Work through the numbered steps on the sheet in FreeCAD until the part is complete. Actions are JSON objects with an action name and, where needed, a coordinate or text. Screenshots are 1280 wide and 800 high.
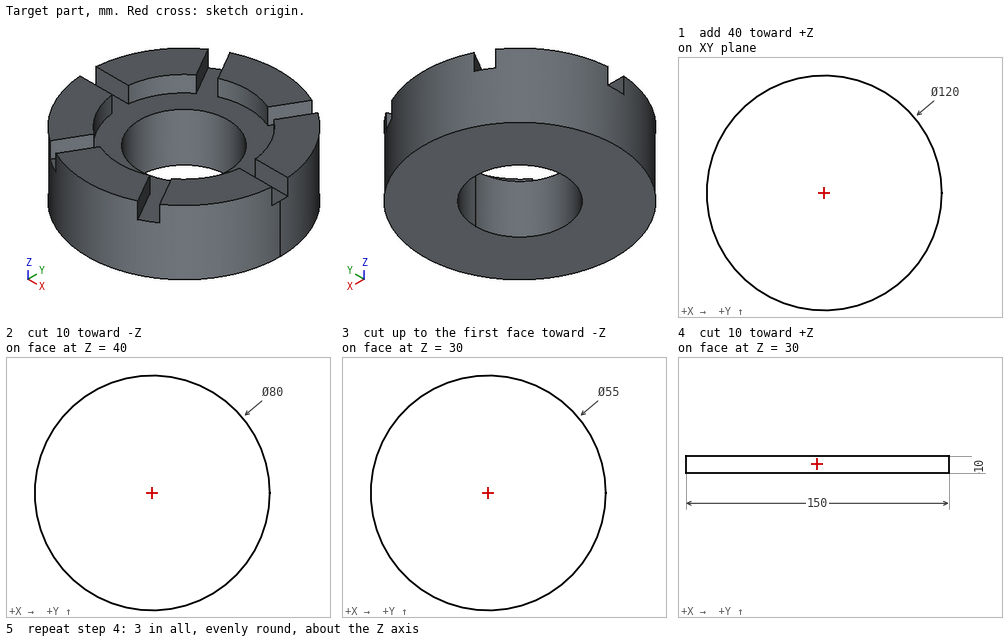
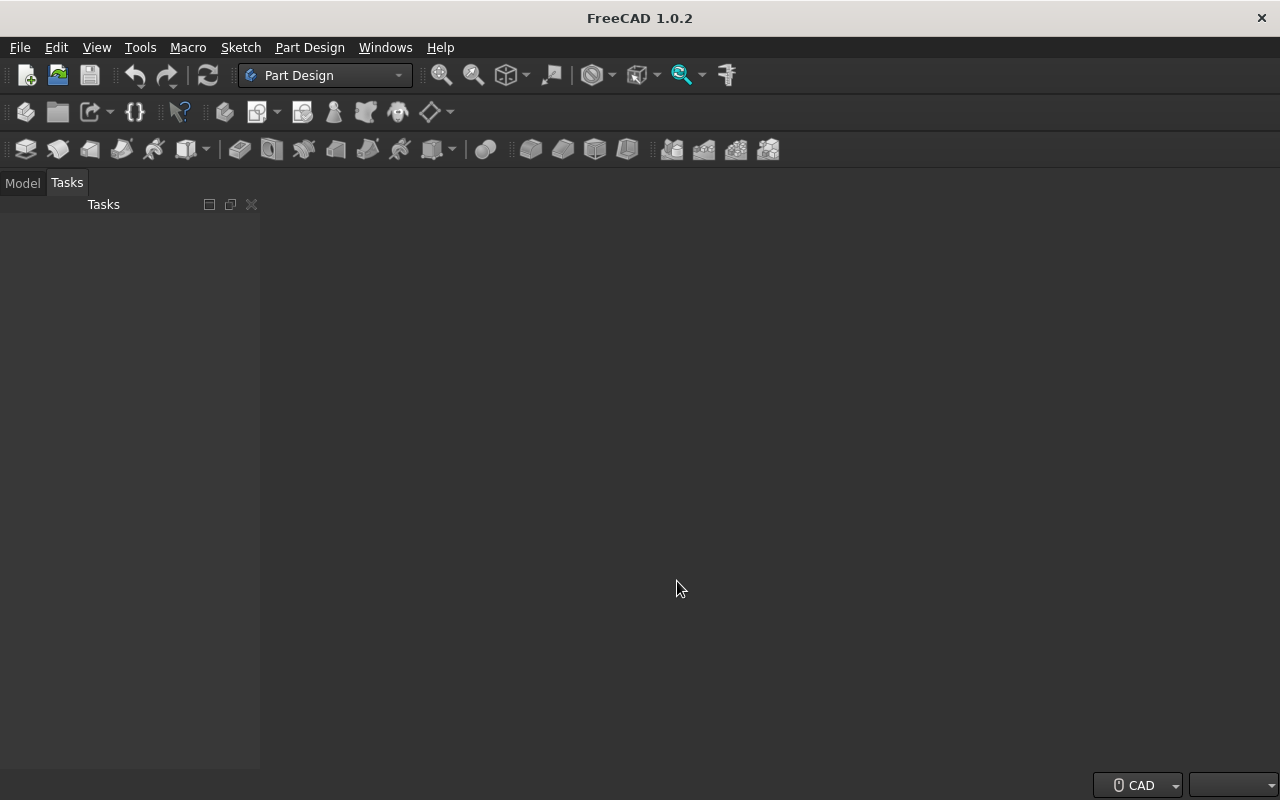
{"action": "left_click", "coordinate": [26, 76]}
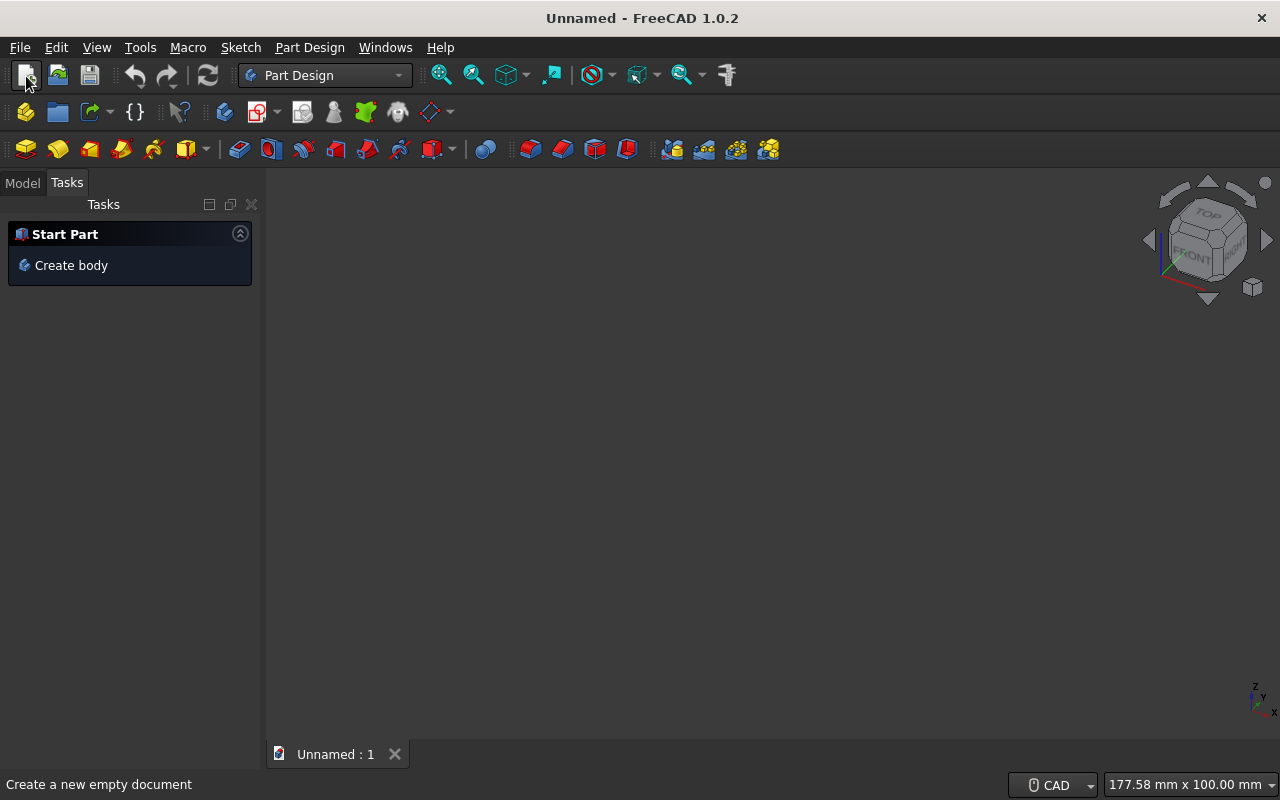
{"action": "left_click", "coordinate": [258, 112]}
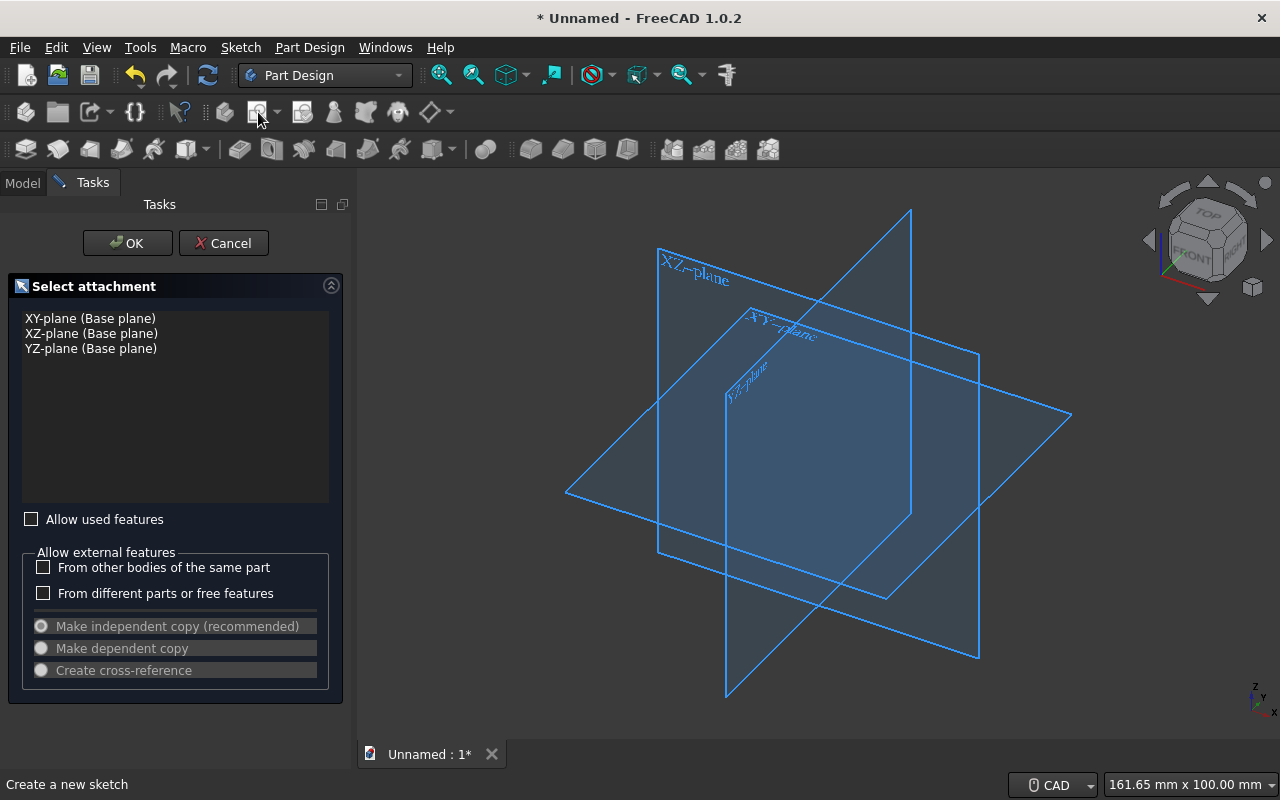
{"action": "left_click", "coordinate": [82, 318]}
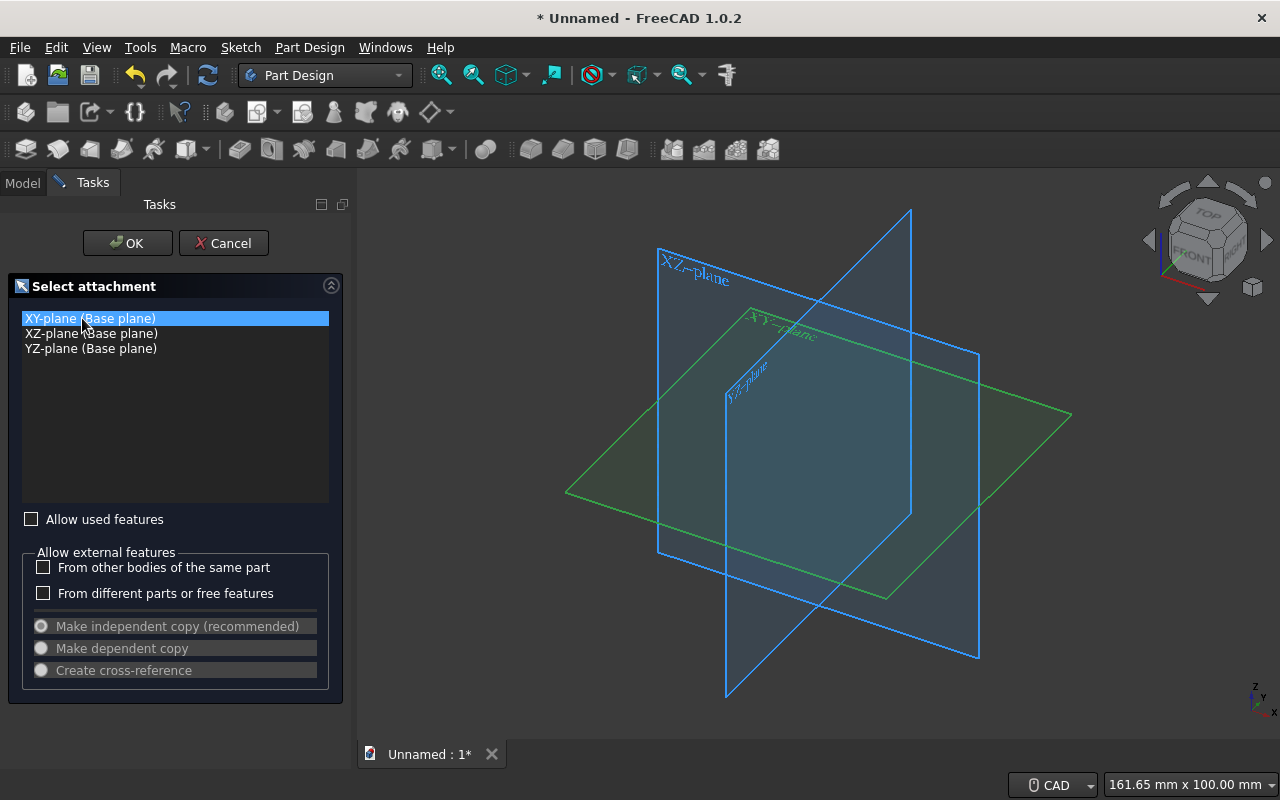
{"action": "left_click", "coordinate": [128, 243]}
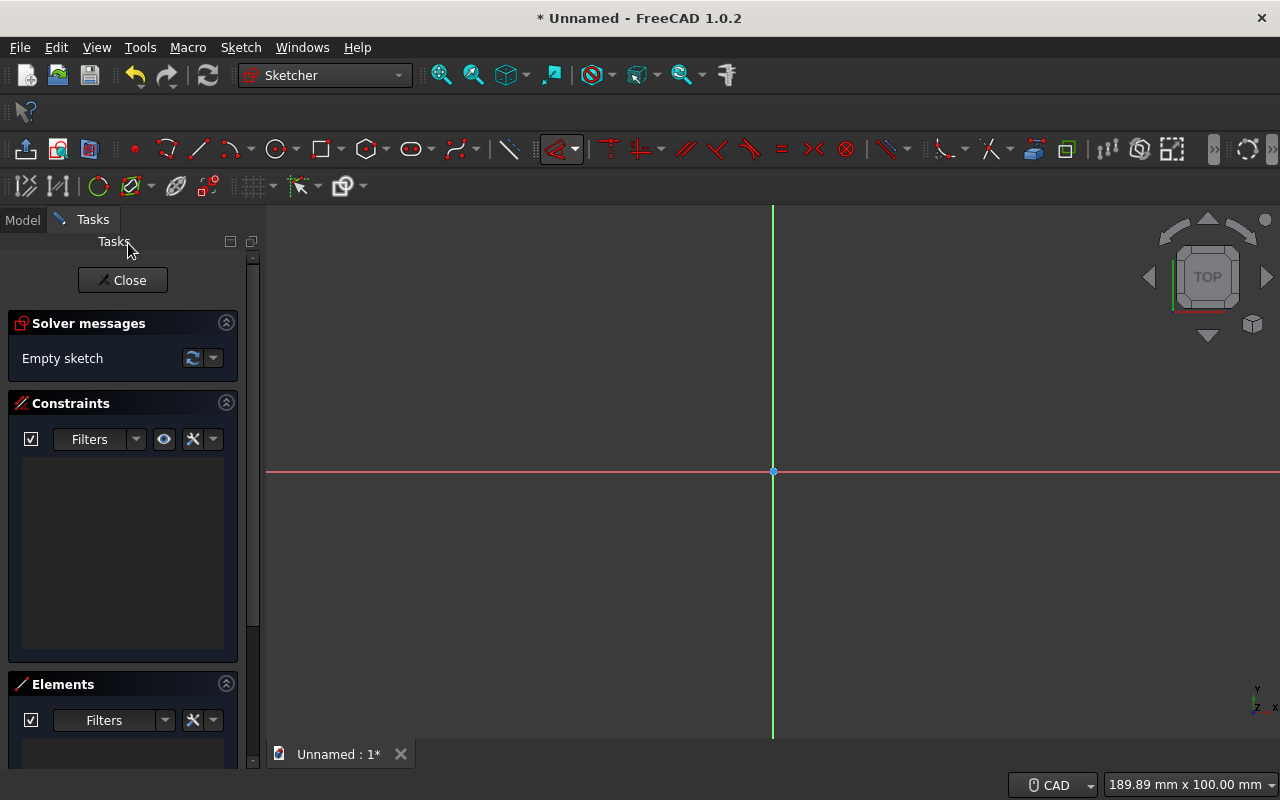
{"action": "scroll", "coordinate": [621, 472], "scroll_direction": "down", "scroll_amount": 3}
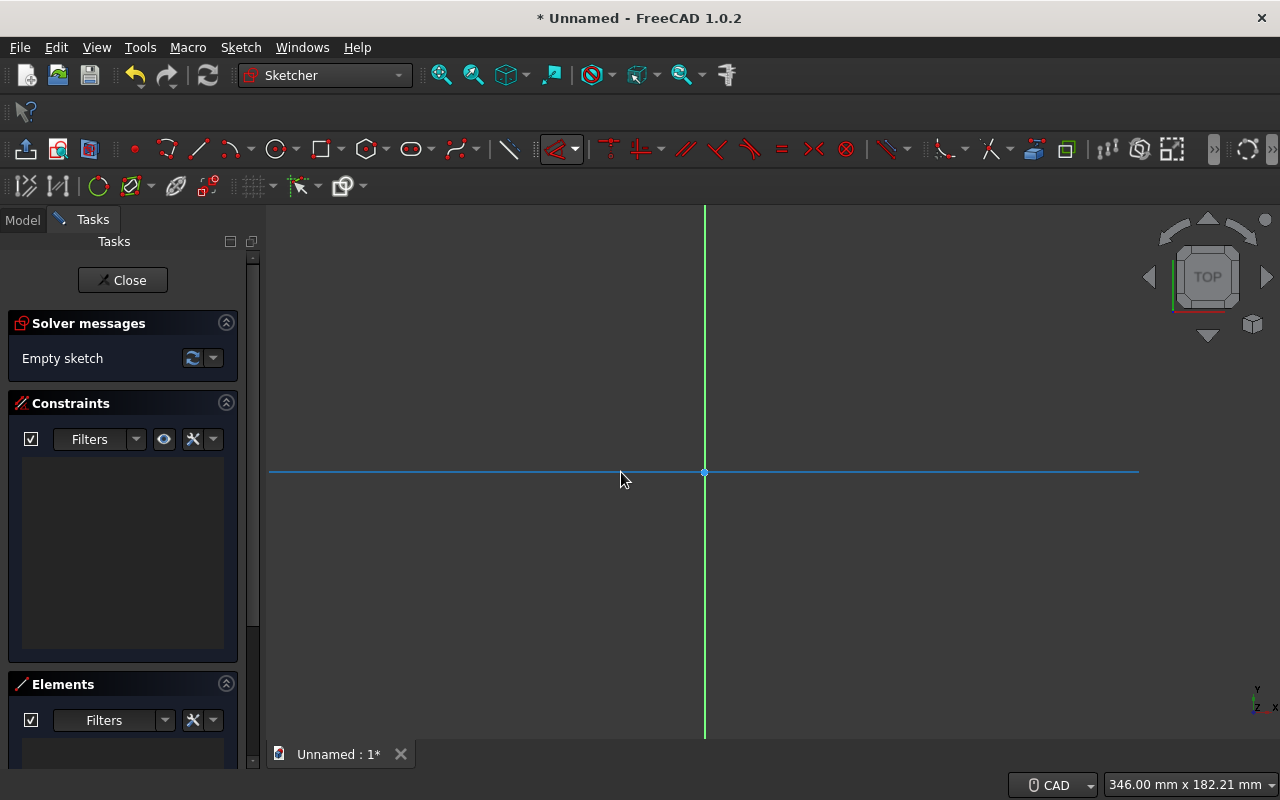
{"action": "left_click", "coordinate": [276, 150]}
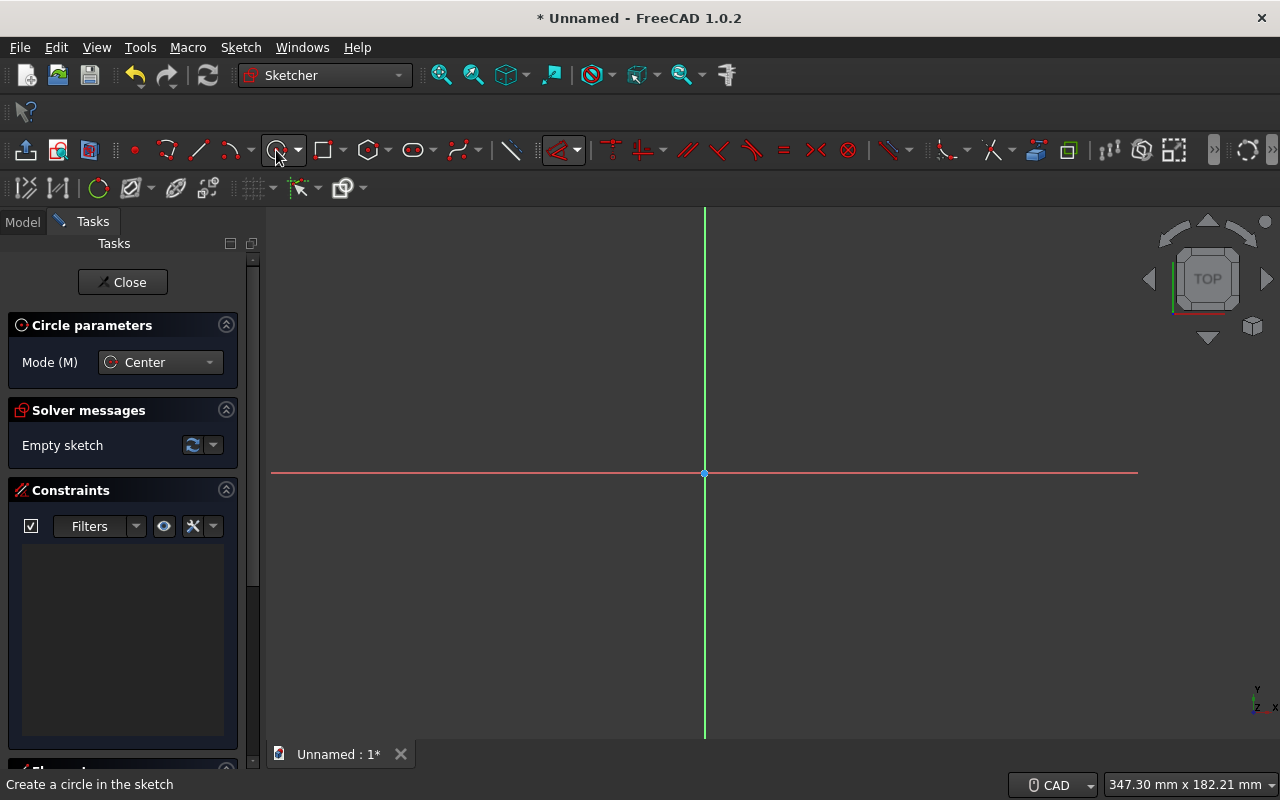
{"action": "left_click", "coordinate": [705, 473]}
{"action": "left_click", "coordinate": [829, 349]}
{"action": "key", "text": "Escape"}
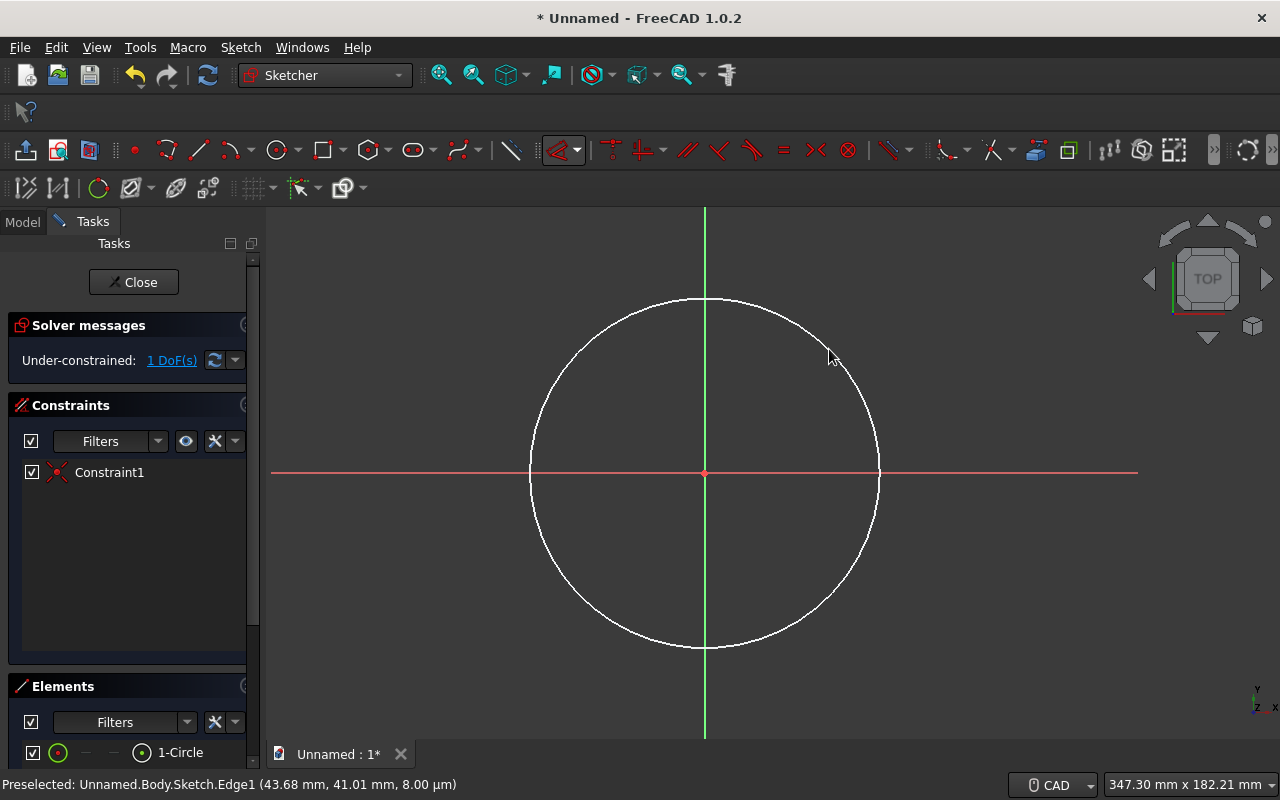
{"action": "key", "text": "d"}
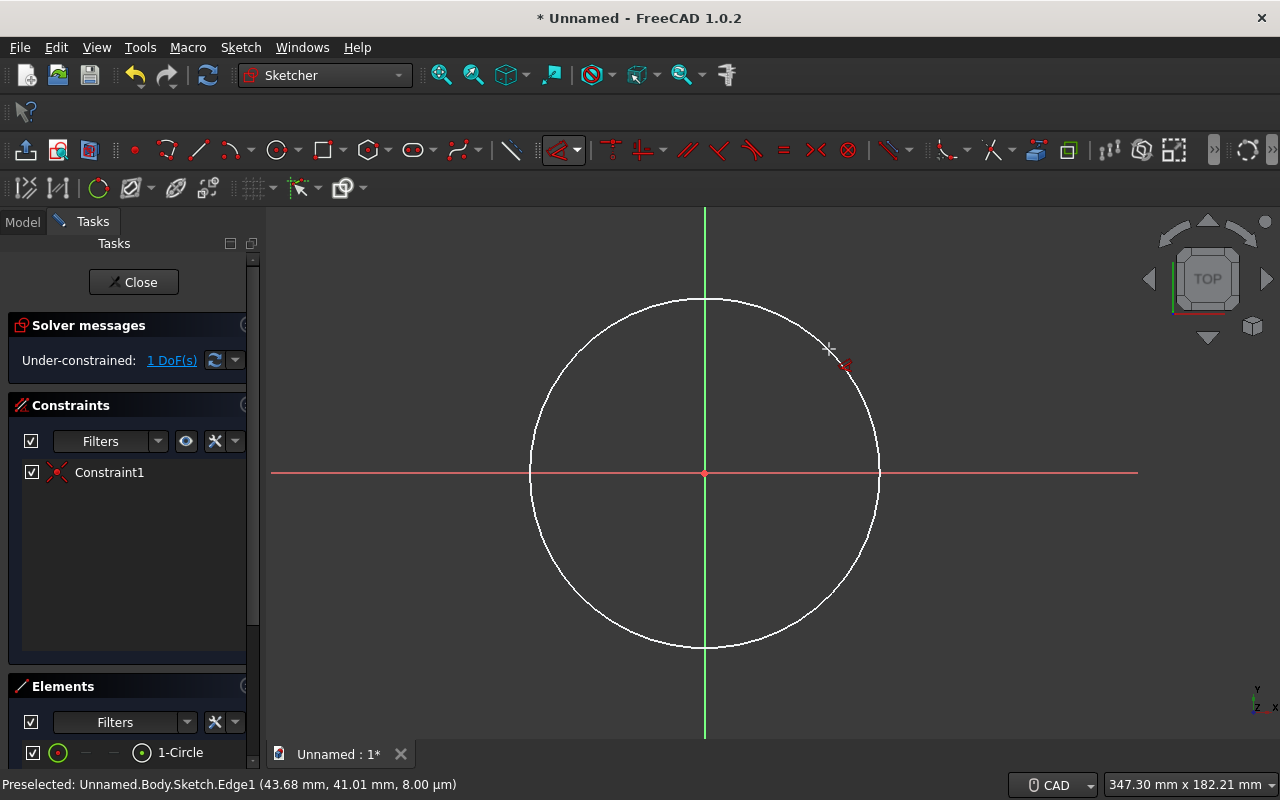
{"action": "left_click", "coordinate": [828, 349]}
{"action": "left_click", "coordinate": [851, 326]}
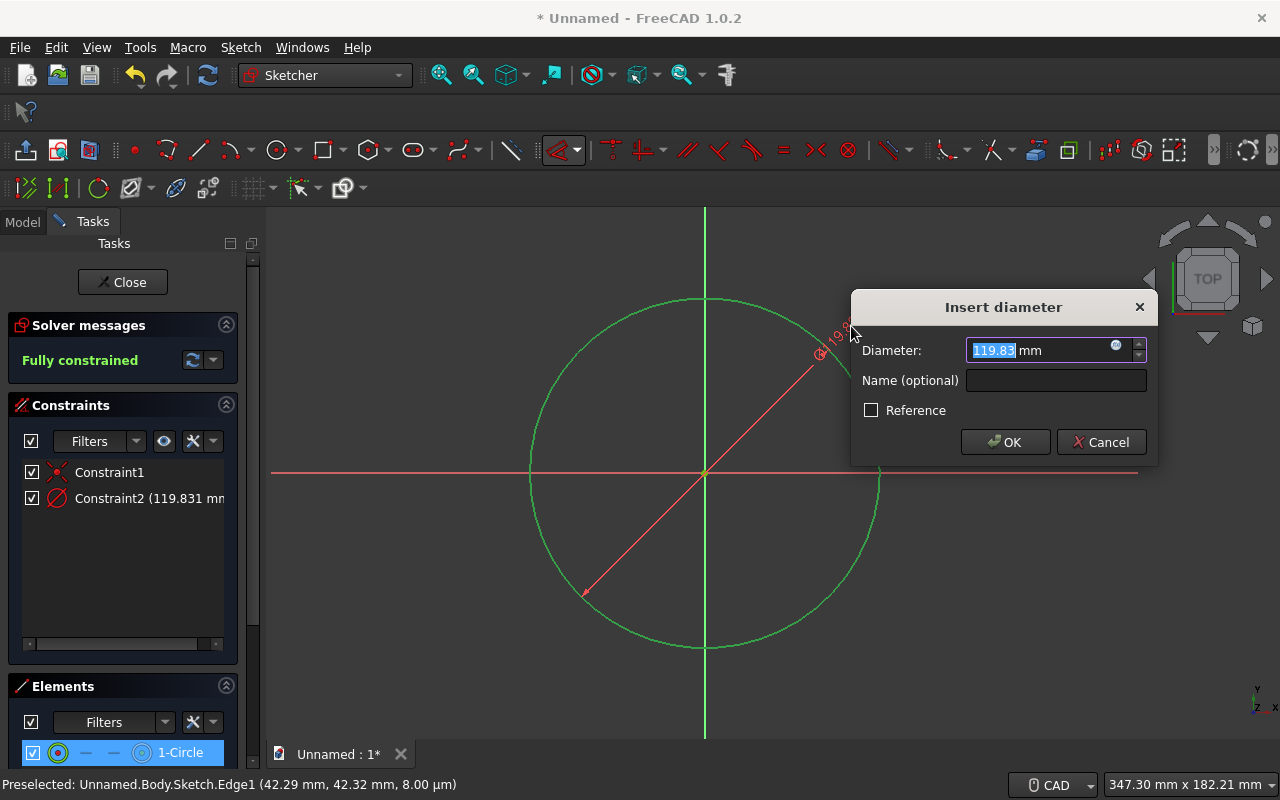
{"action": "type", "text": "120"}
{"action": "key", "text": "Return"}
{"action": "key", "text": "Escape"}